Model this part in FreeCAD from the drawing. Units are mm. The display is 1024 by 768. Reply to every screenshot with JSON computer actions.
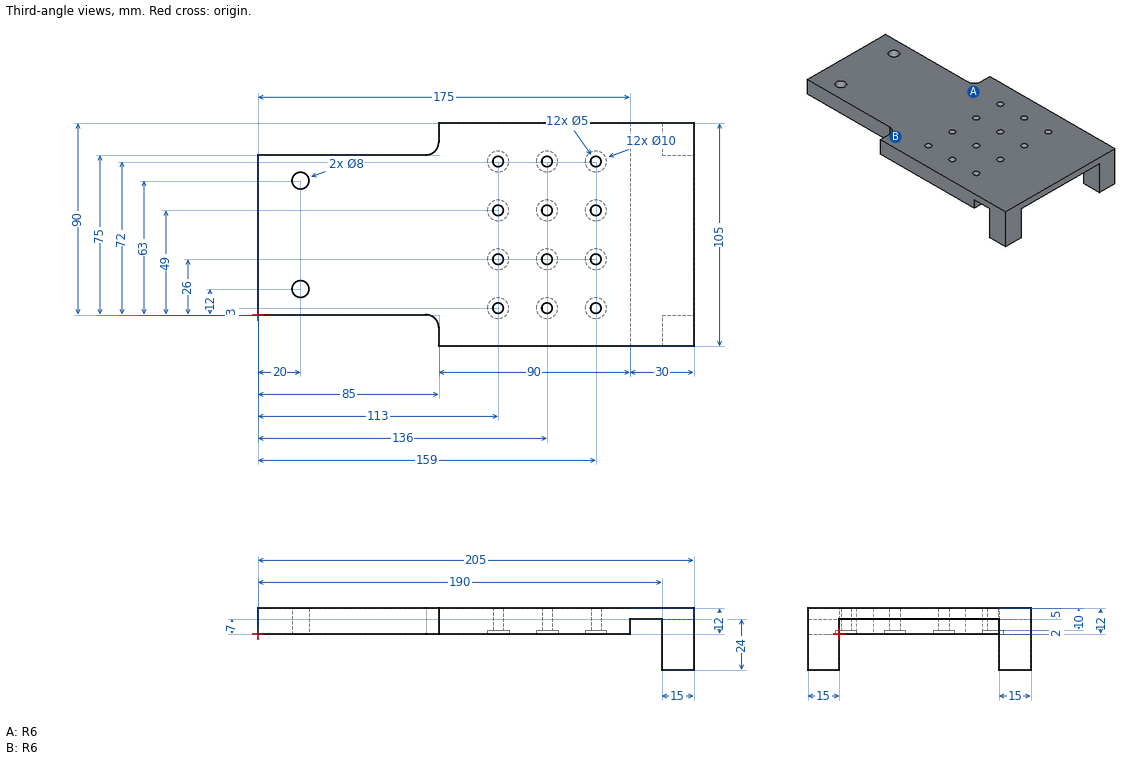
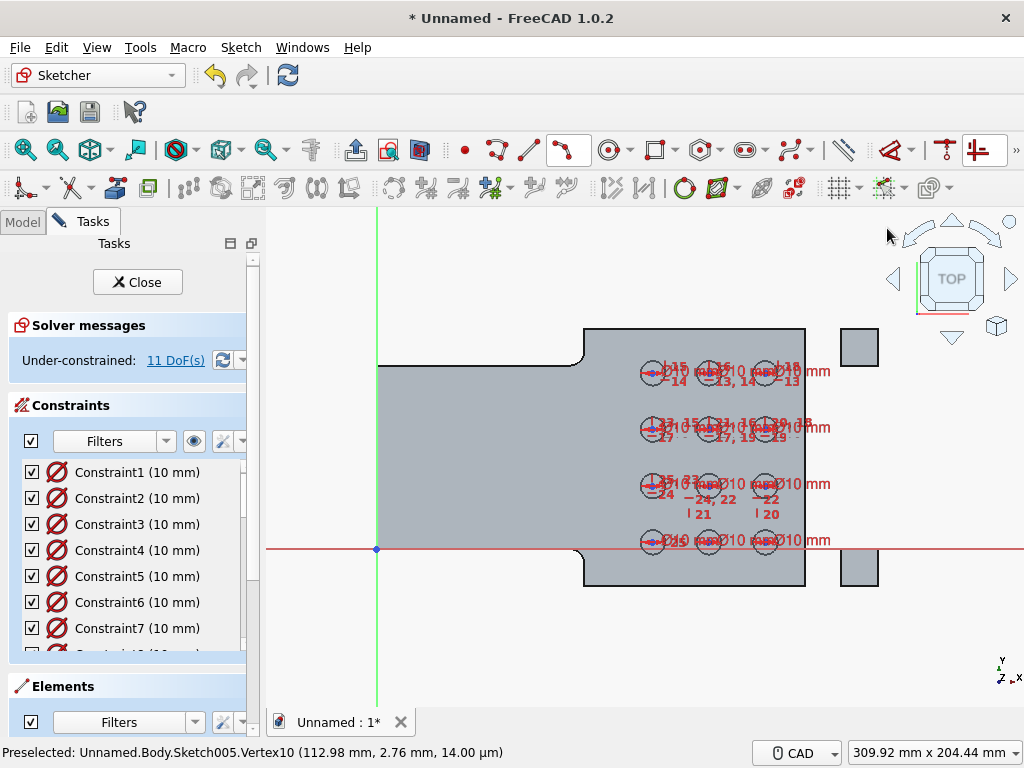
{"action": "left_click", "coordinate": [709, 486]}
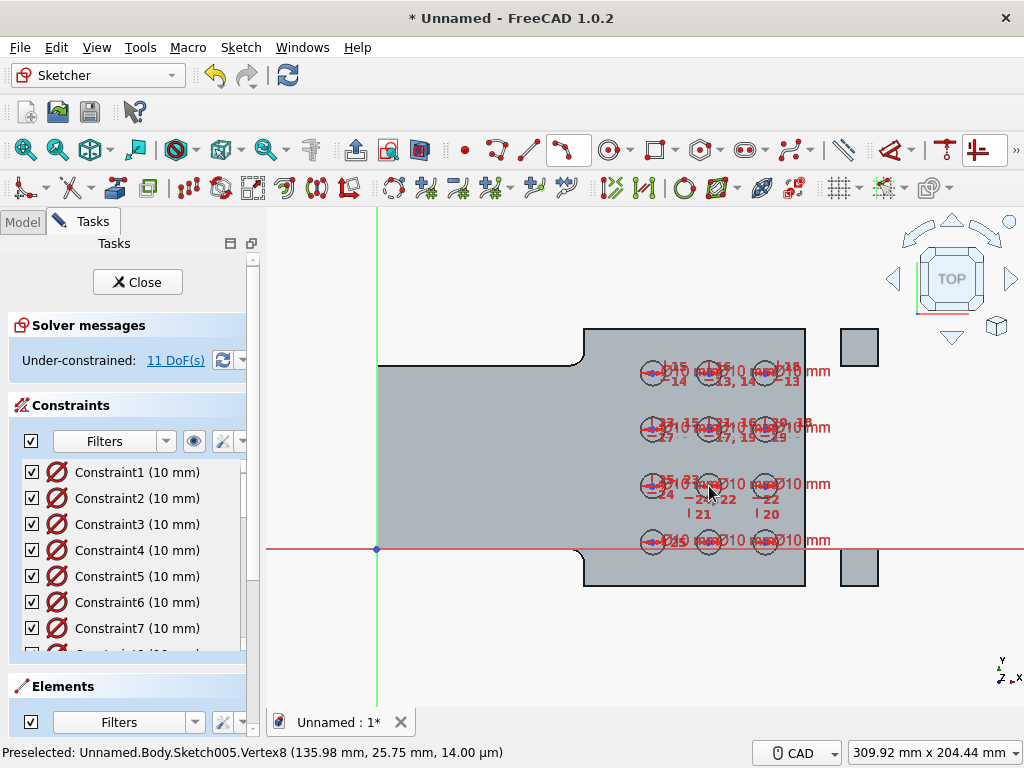
{"action": "left_click", "coordinate": [709, 542]}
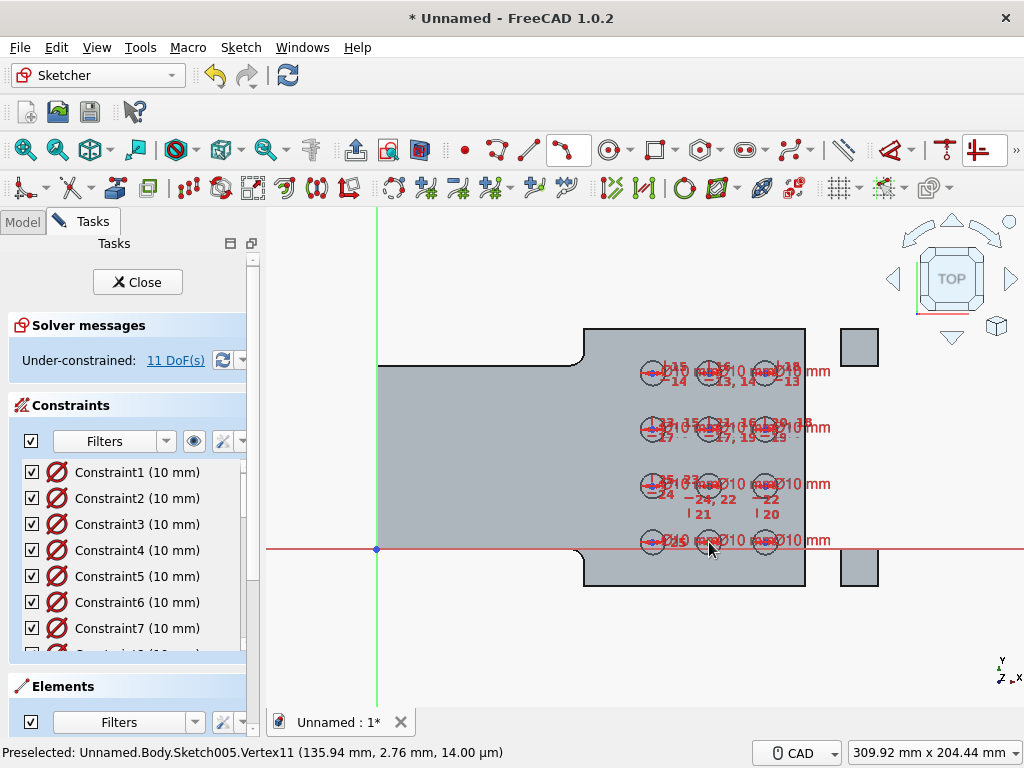
{"action": "key", "text": "v"}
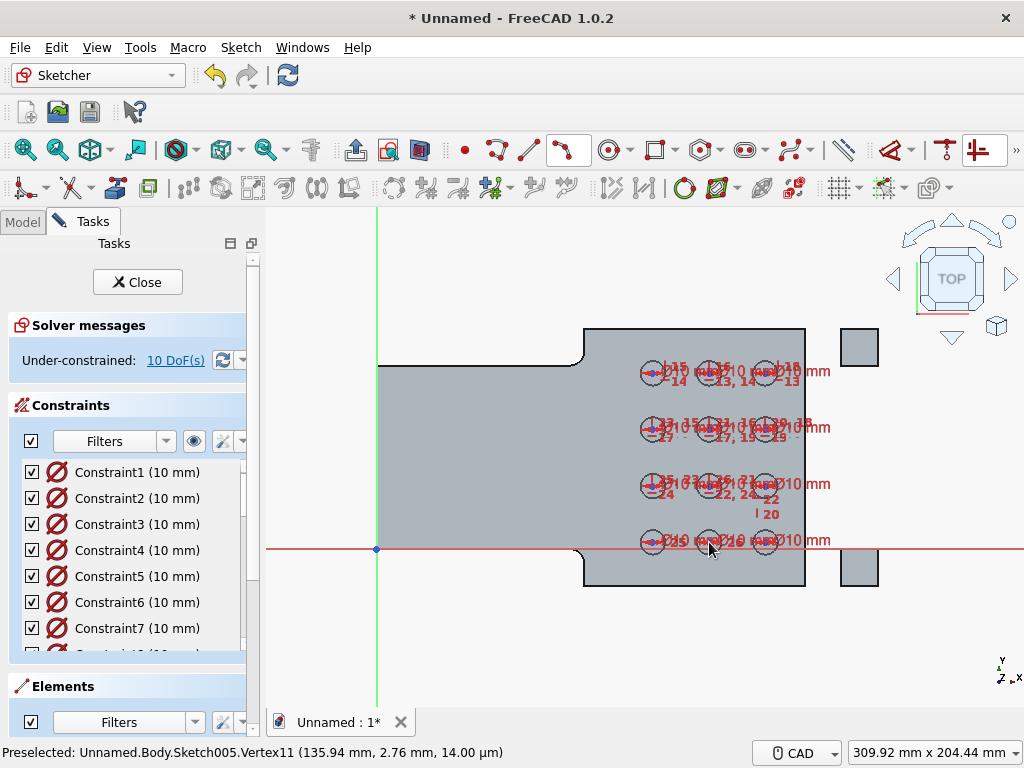
{"action": "left_click", "coordinate": [653, 542]}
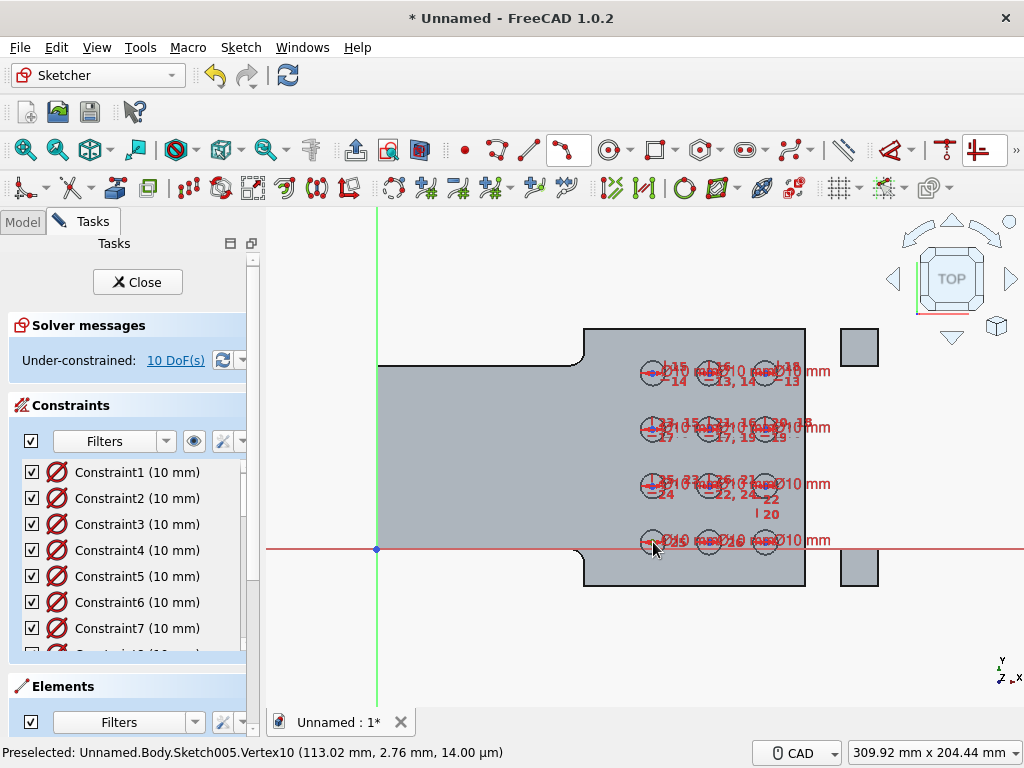
{"action": "left_click", "coordinate": [709, 542]}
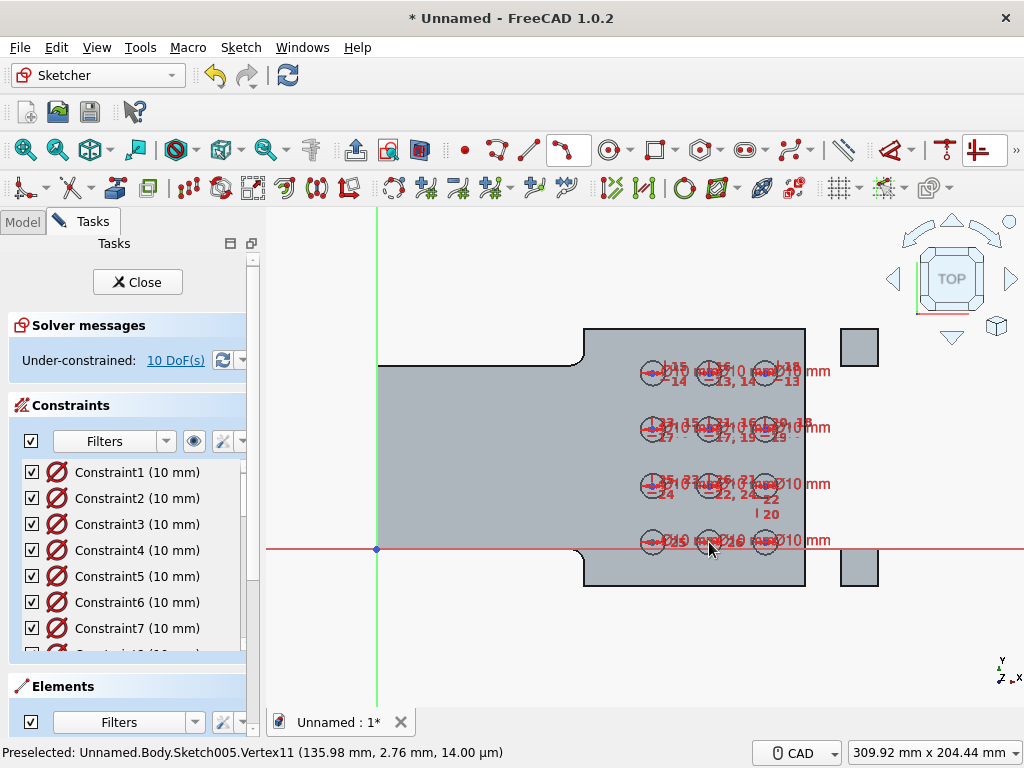
{"action": "key", "text": "h"}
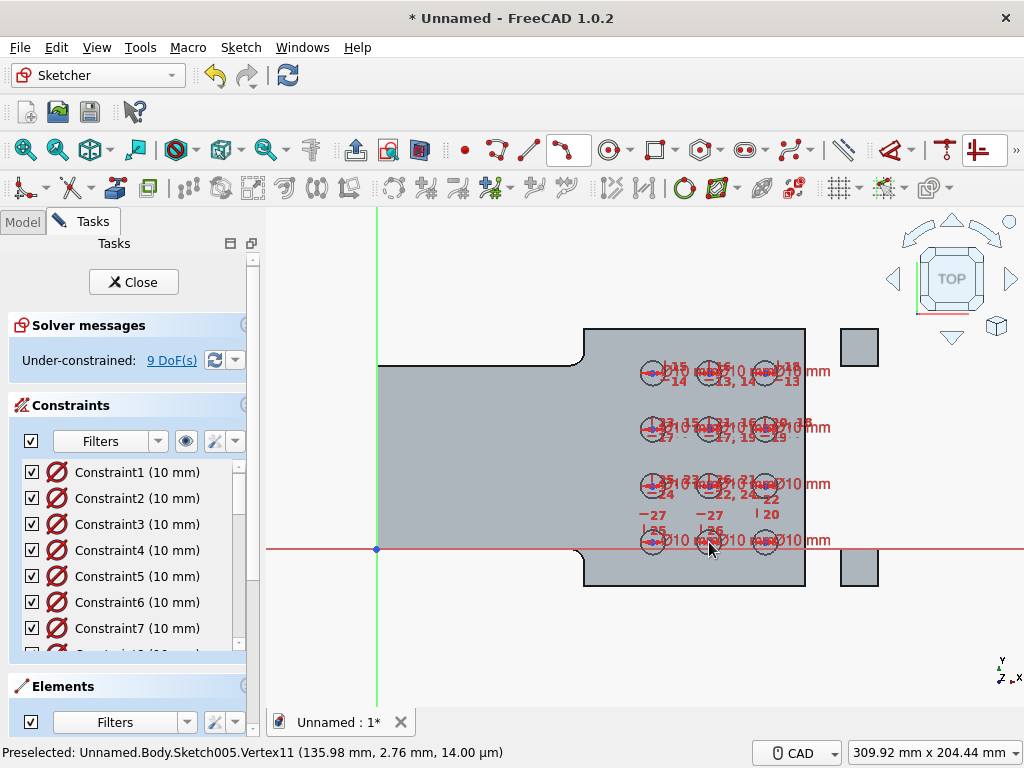
{"action": "left_click", "coordinate": [765, 486]}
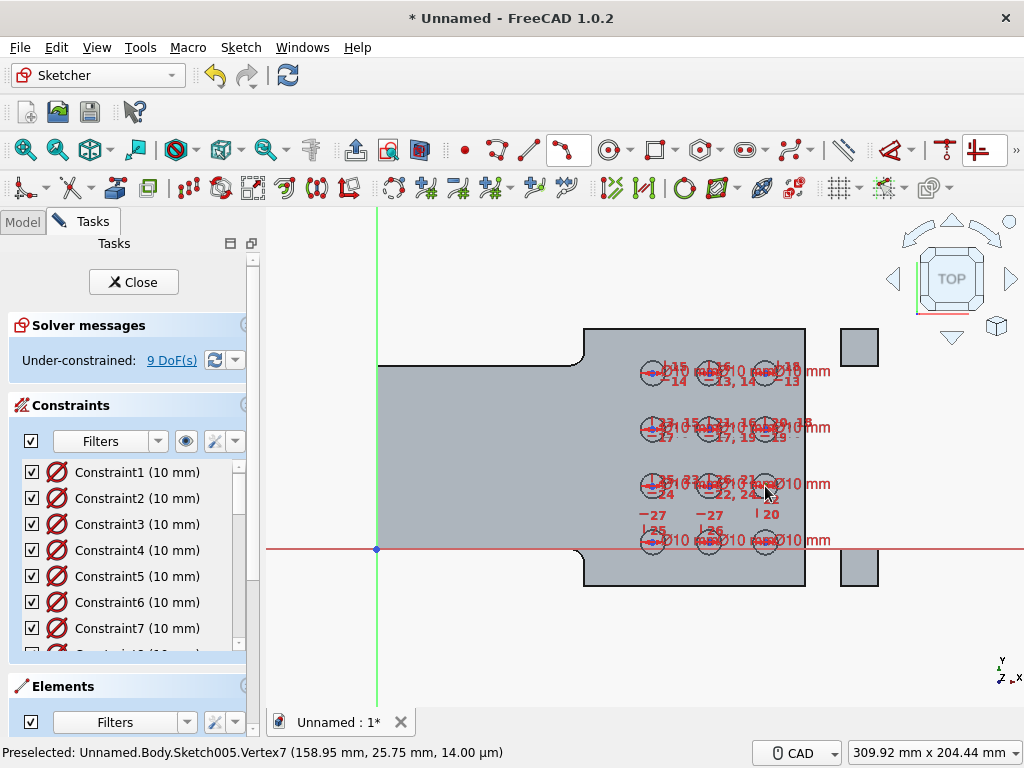
{"action": "left_click", "coordinate": [765, 542]}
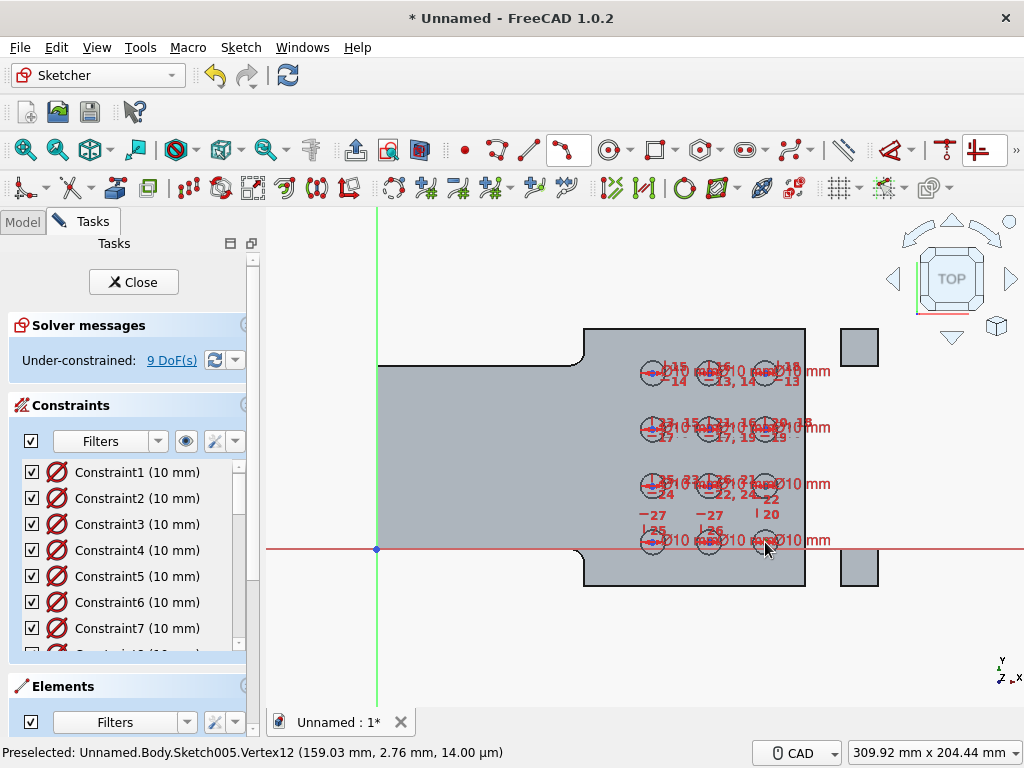
{"action": "key", "text": "v"}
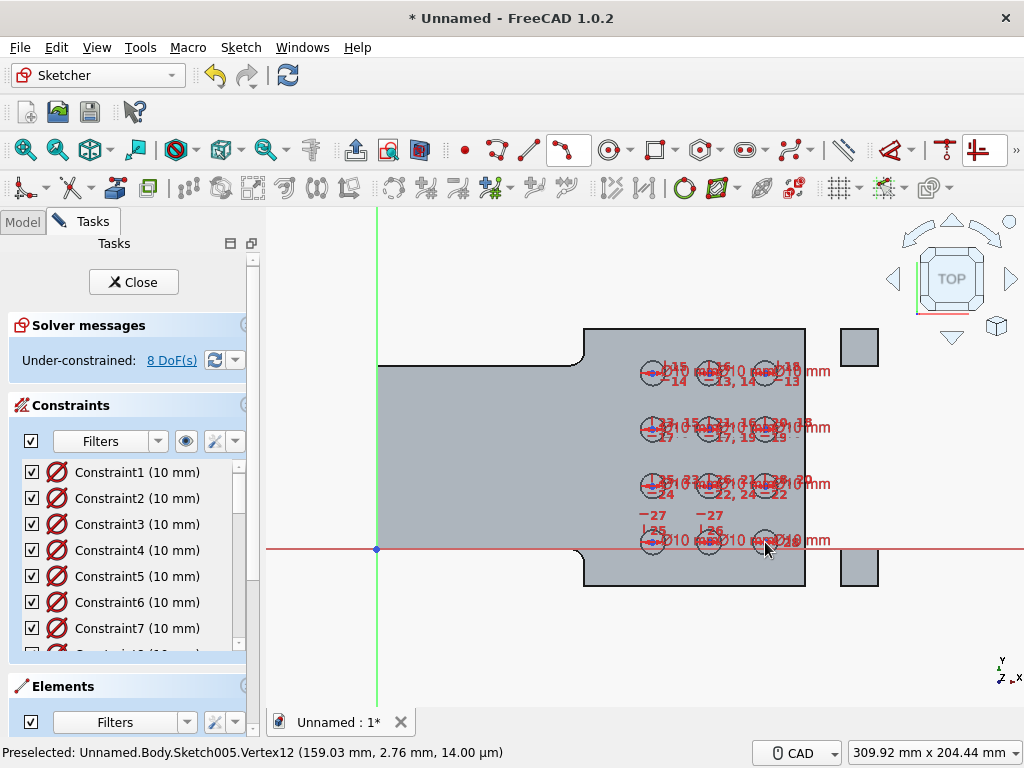
{"action": "left_click", "coordinate": [709, 542]}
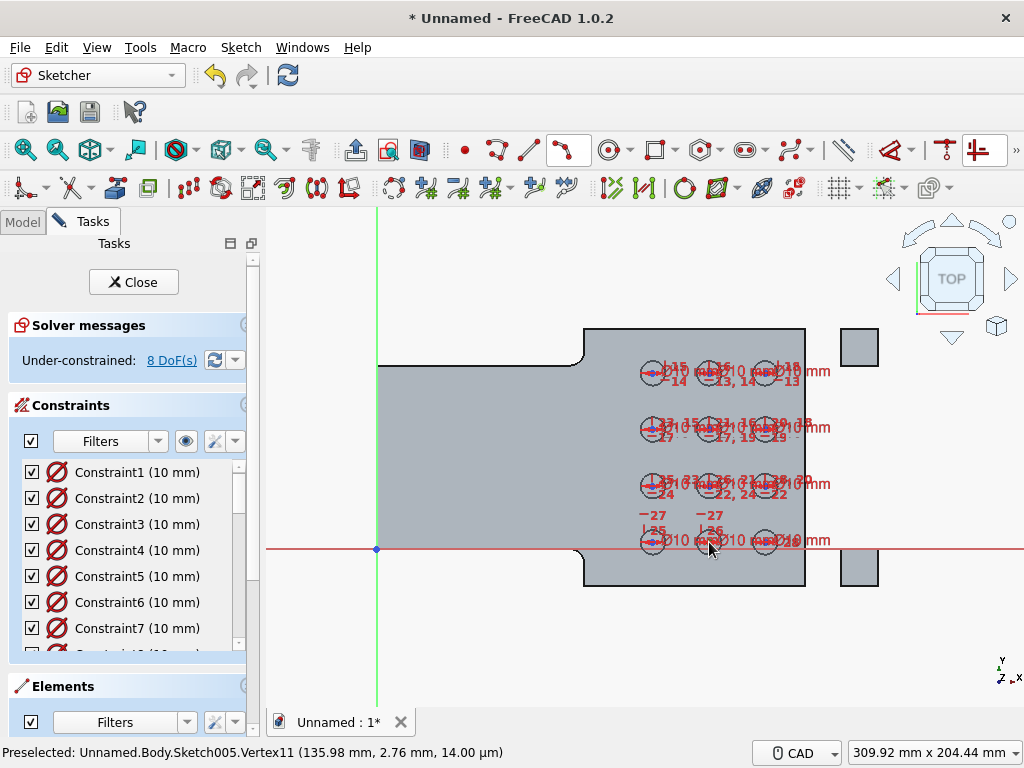
{"action": "left_click", "coordinate": [765, 542]}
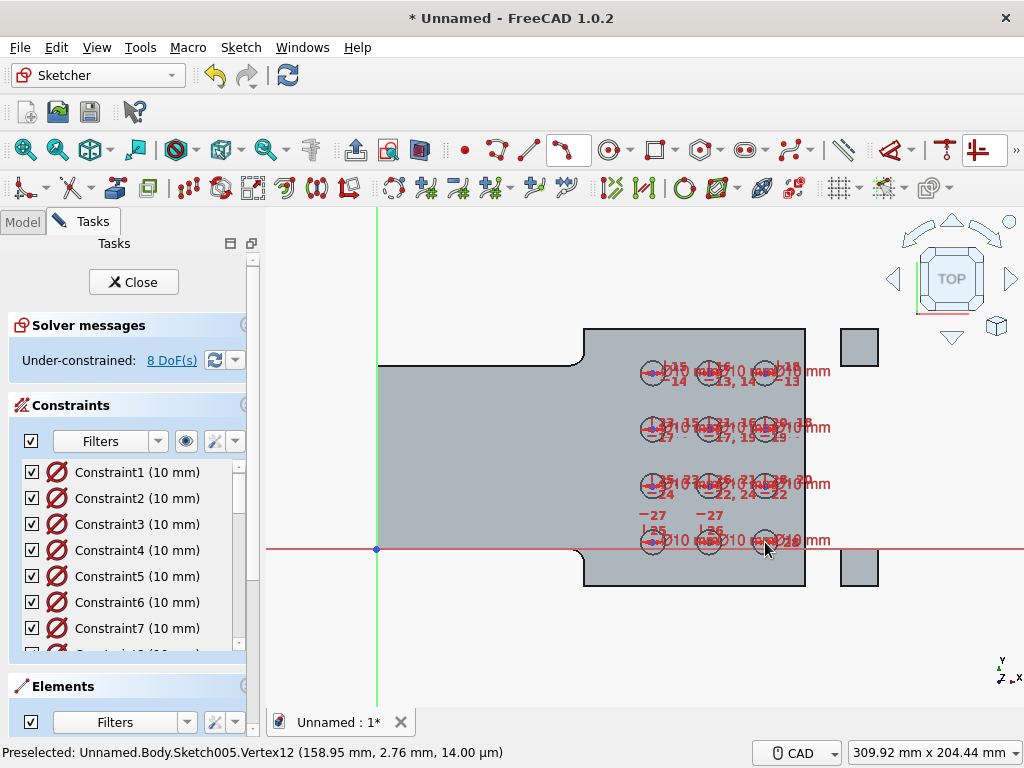
{"action": "left_click", "coordinate": [1002, 150]}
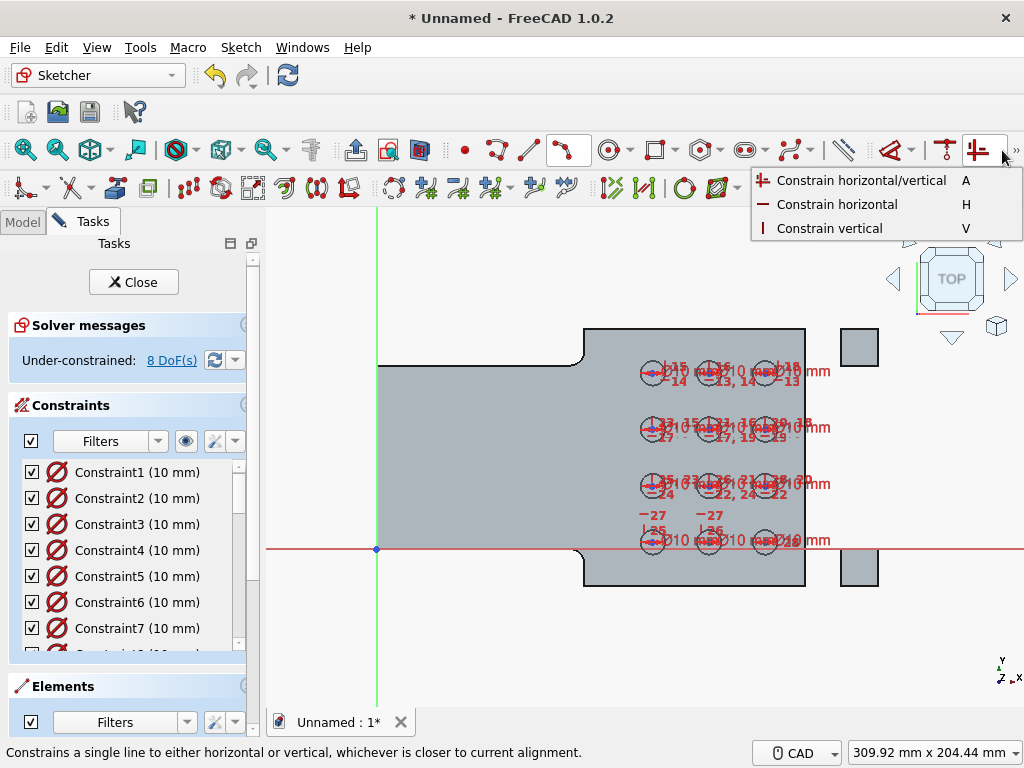
{"action": "left_click", "coordinate": [887, 204]}